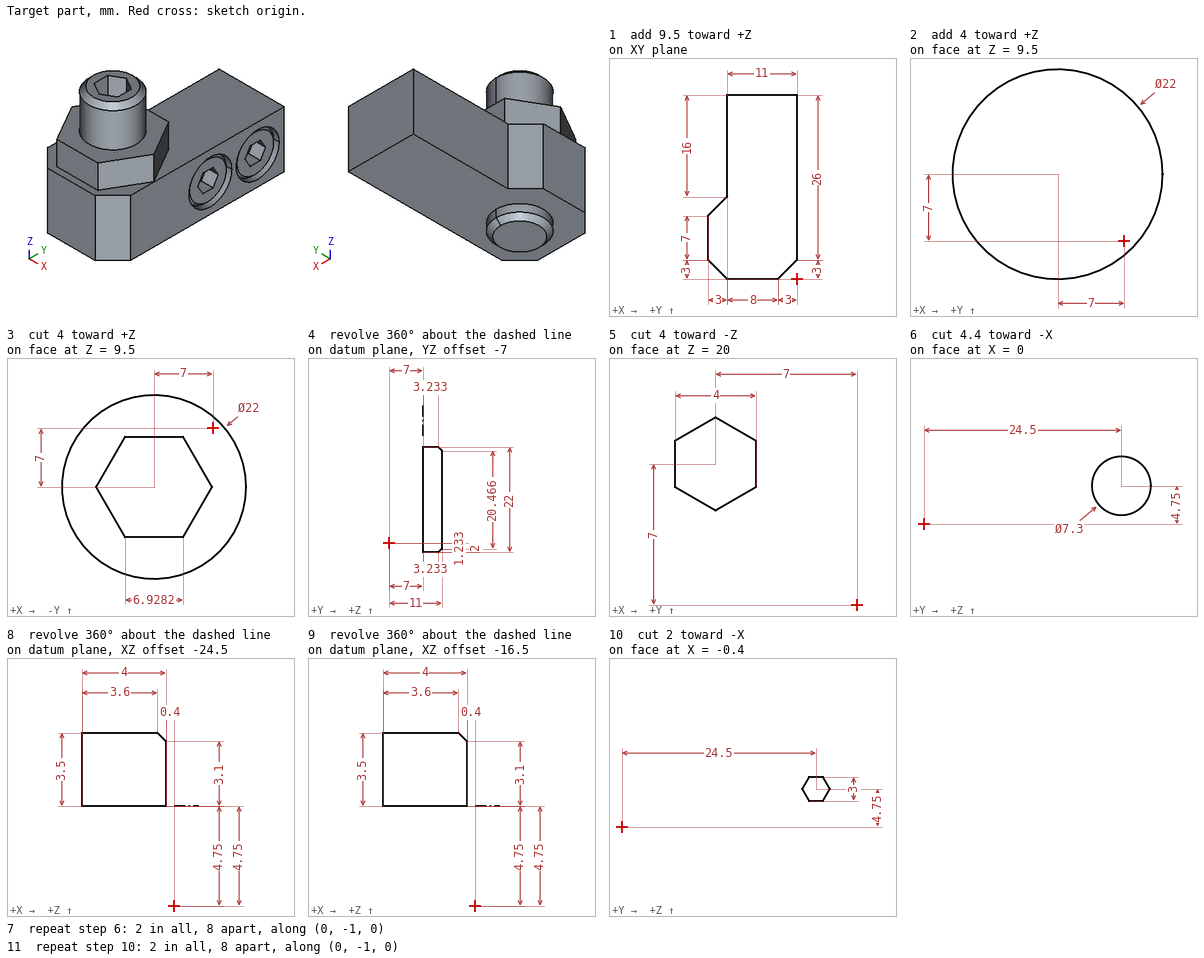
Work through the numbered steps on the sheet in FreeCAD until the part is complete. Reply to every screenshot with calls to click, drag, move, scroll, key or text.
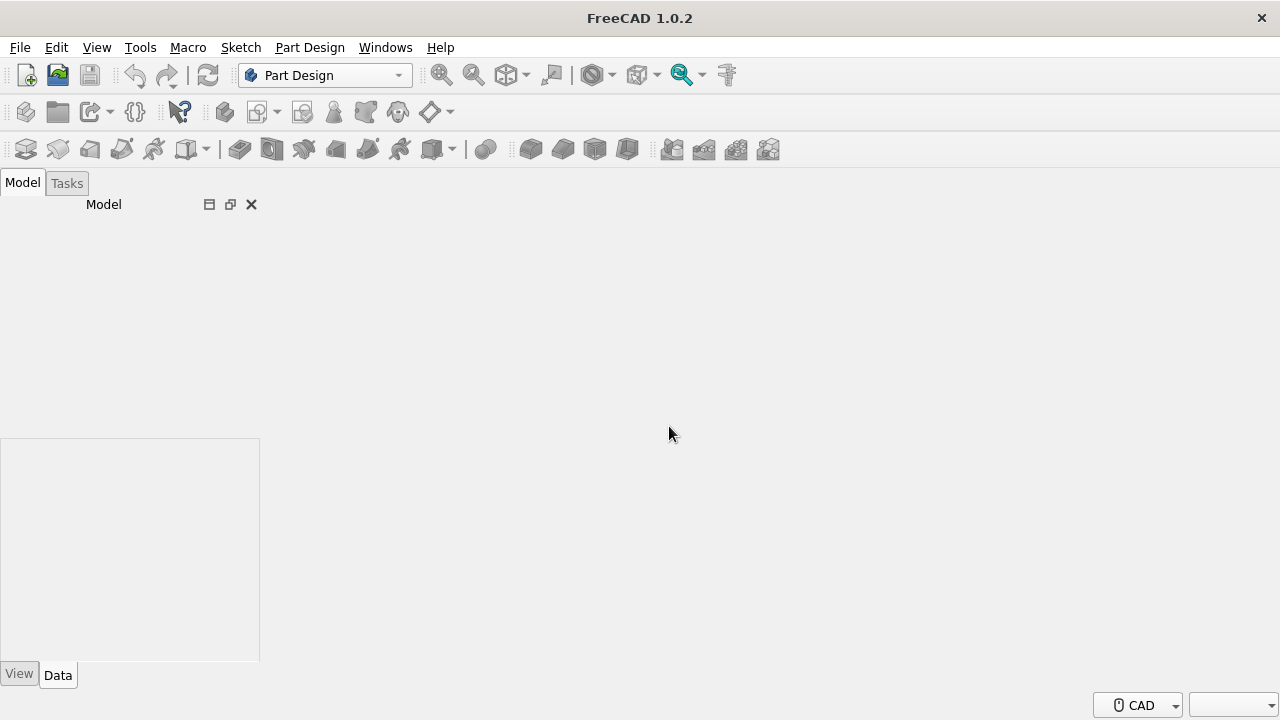
click(26, 76)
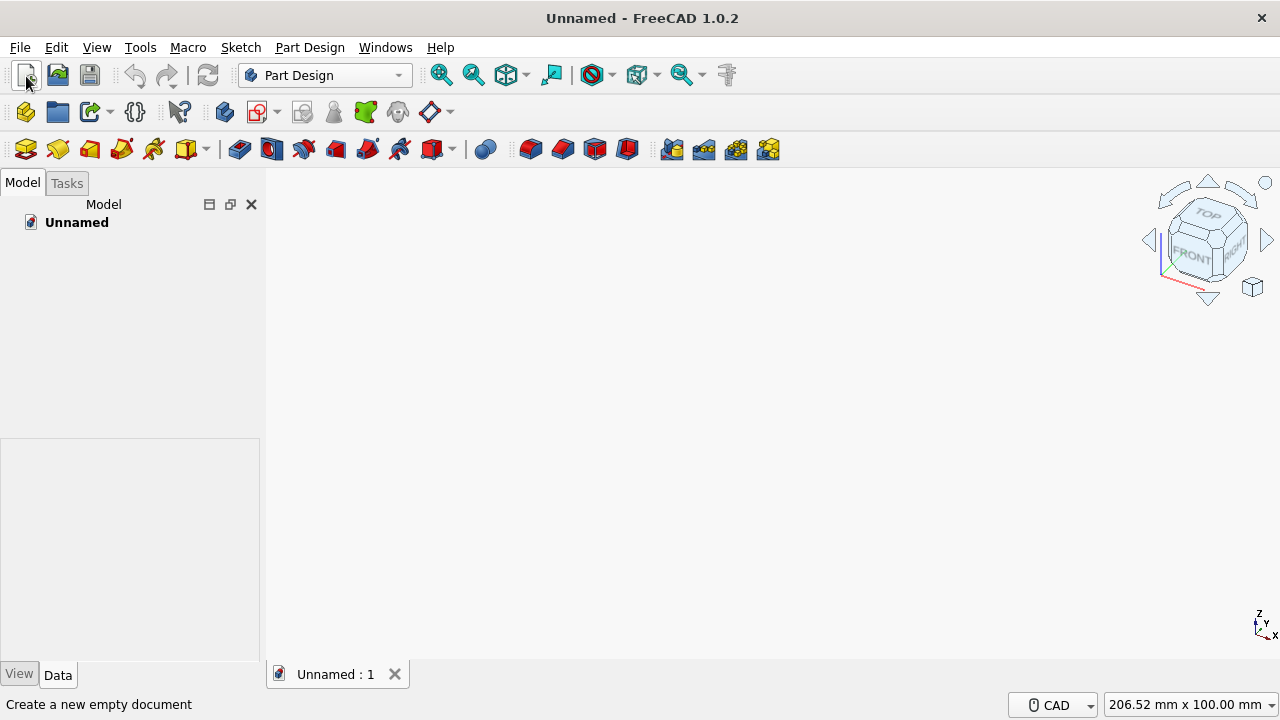
click(258, 112)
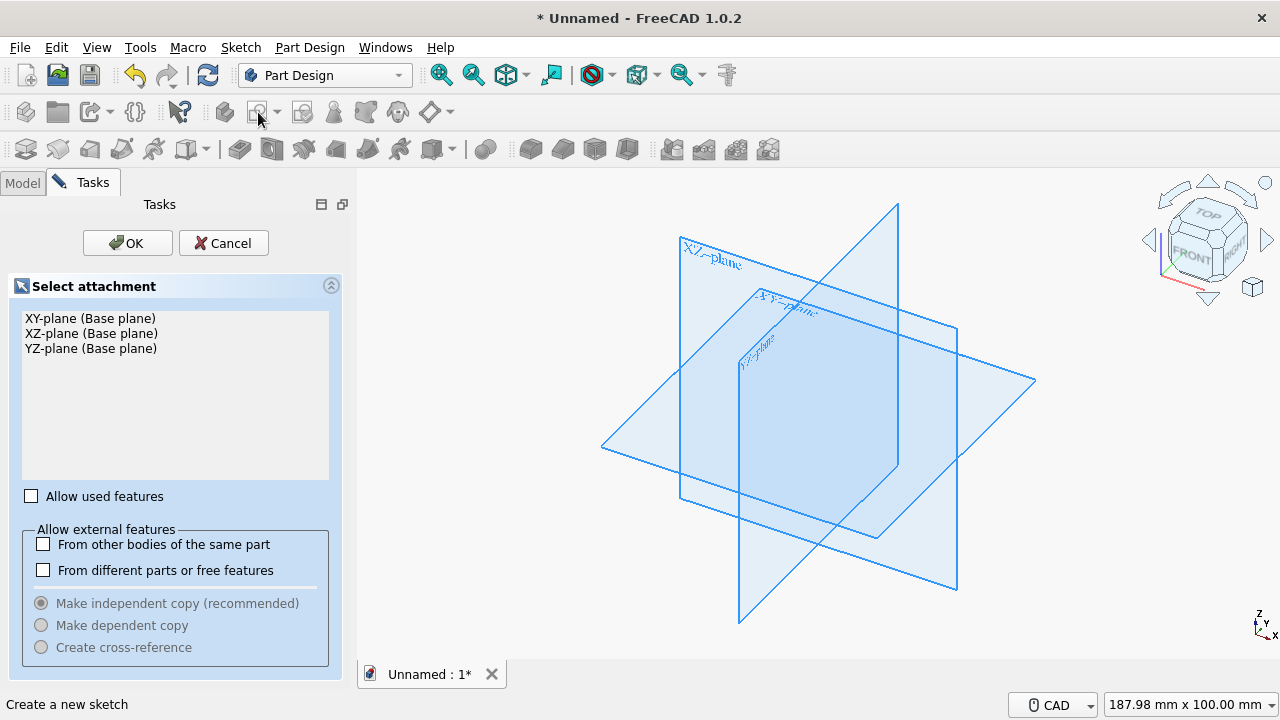
click(82, 318)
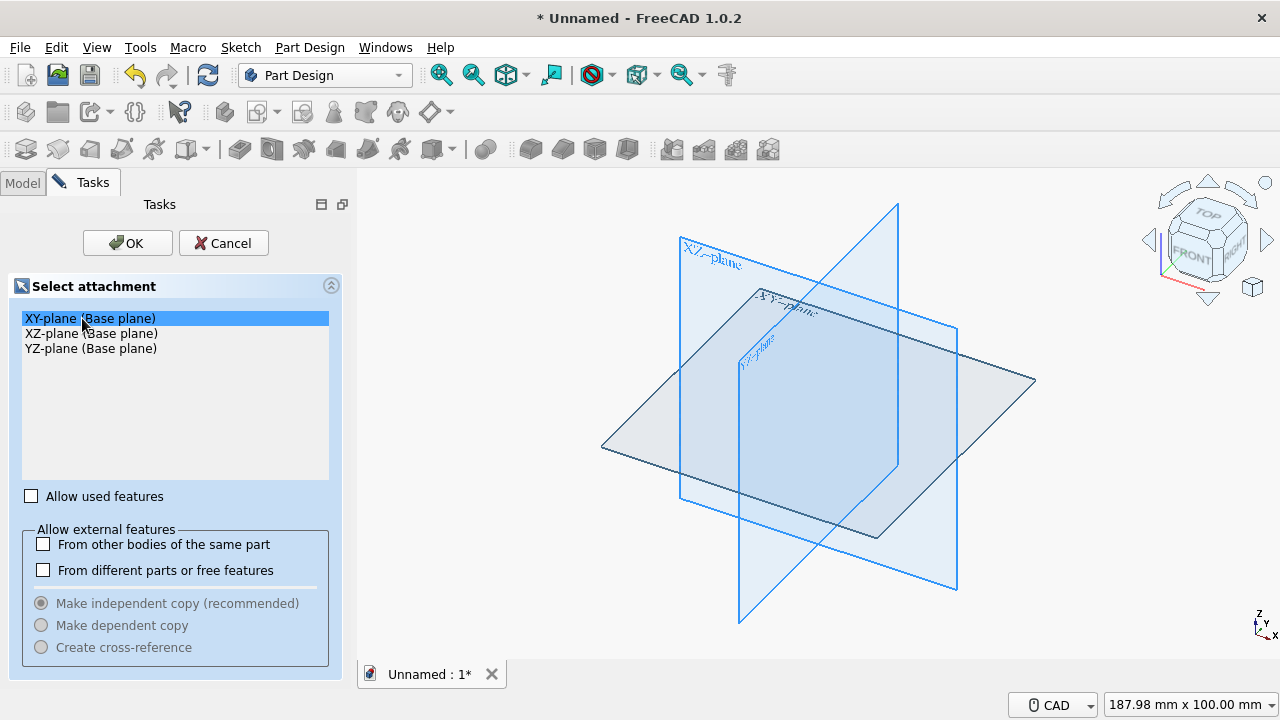
click(128, 243)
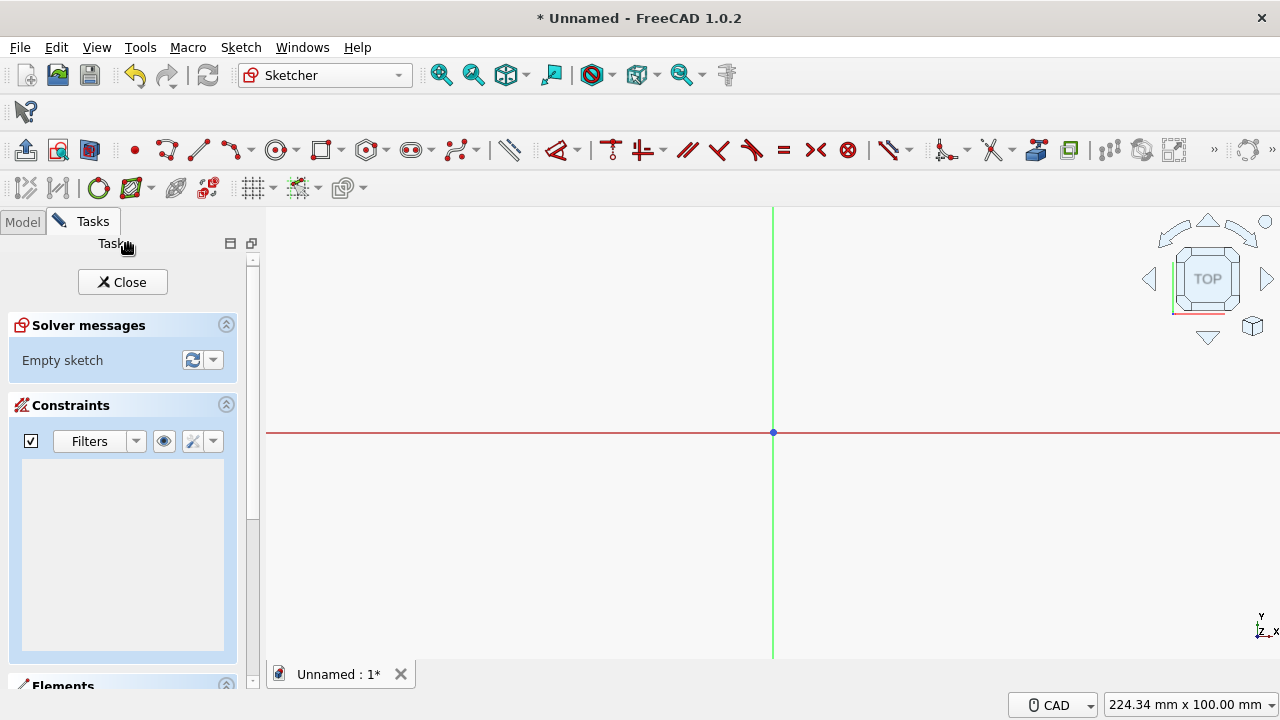
scroll(771, 314, up, 4)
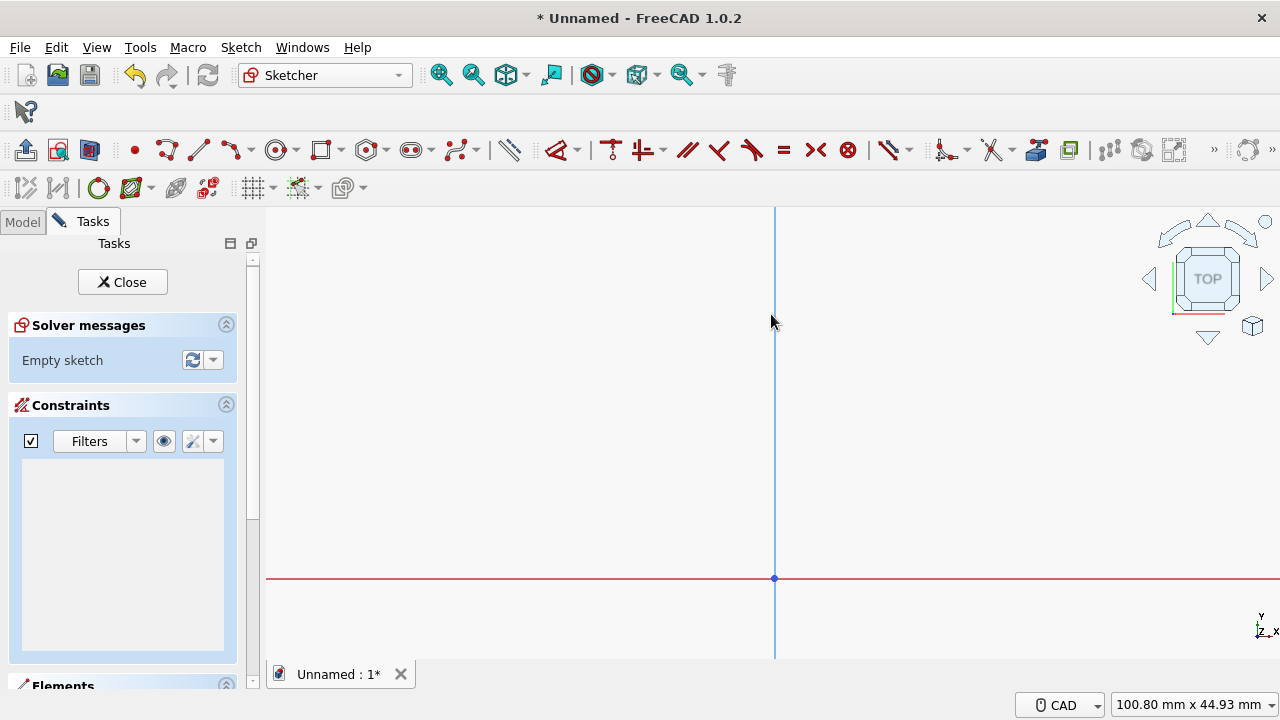
key(g)
key(m)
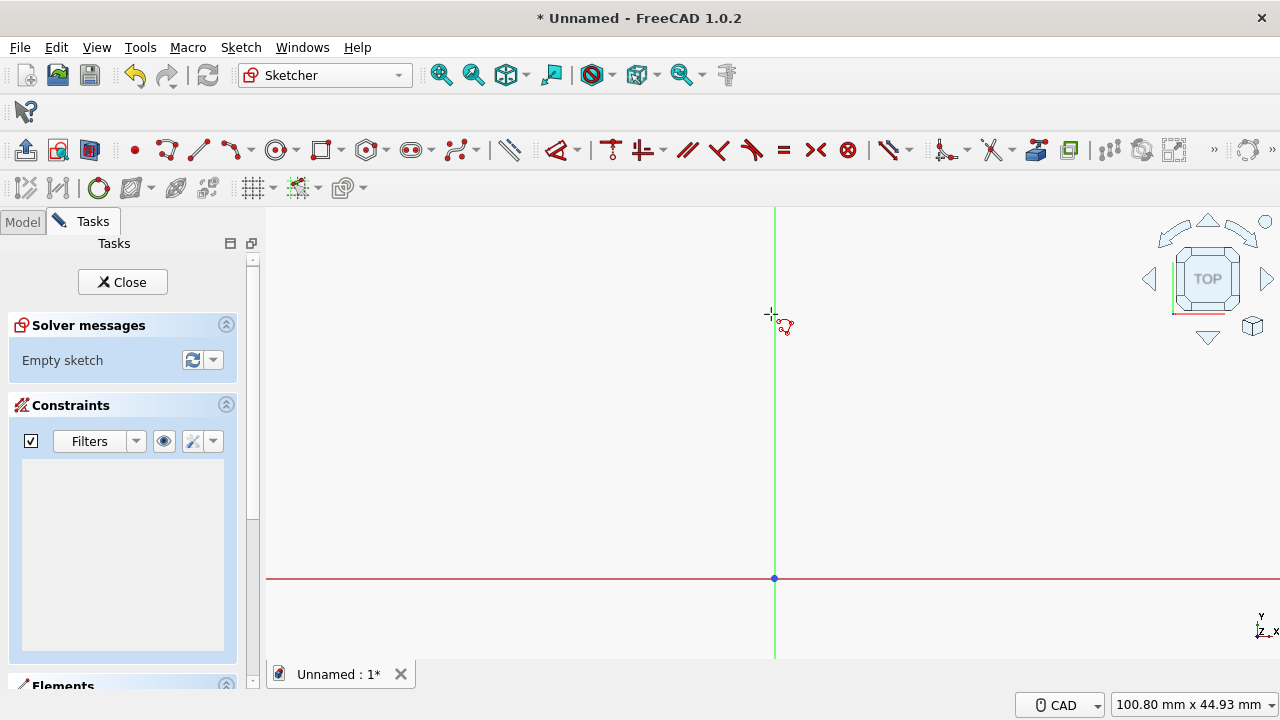
click(745, 579)
click(775, 548)
click(766, 287)
click(664, 287)
click(664, 448)
click(634, 478)
click(634, 548)
click(664, 570)
click(745, 579)
key(Escape)
key(Escape)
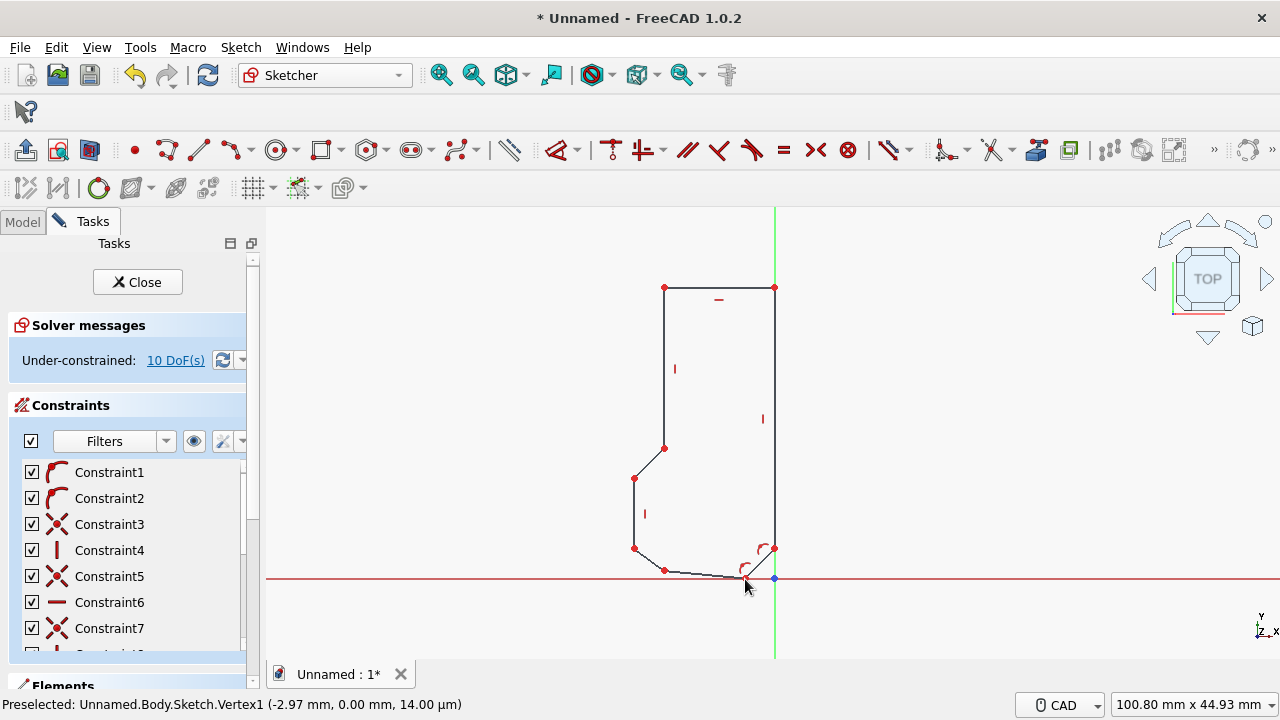
click(721, 576)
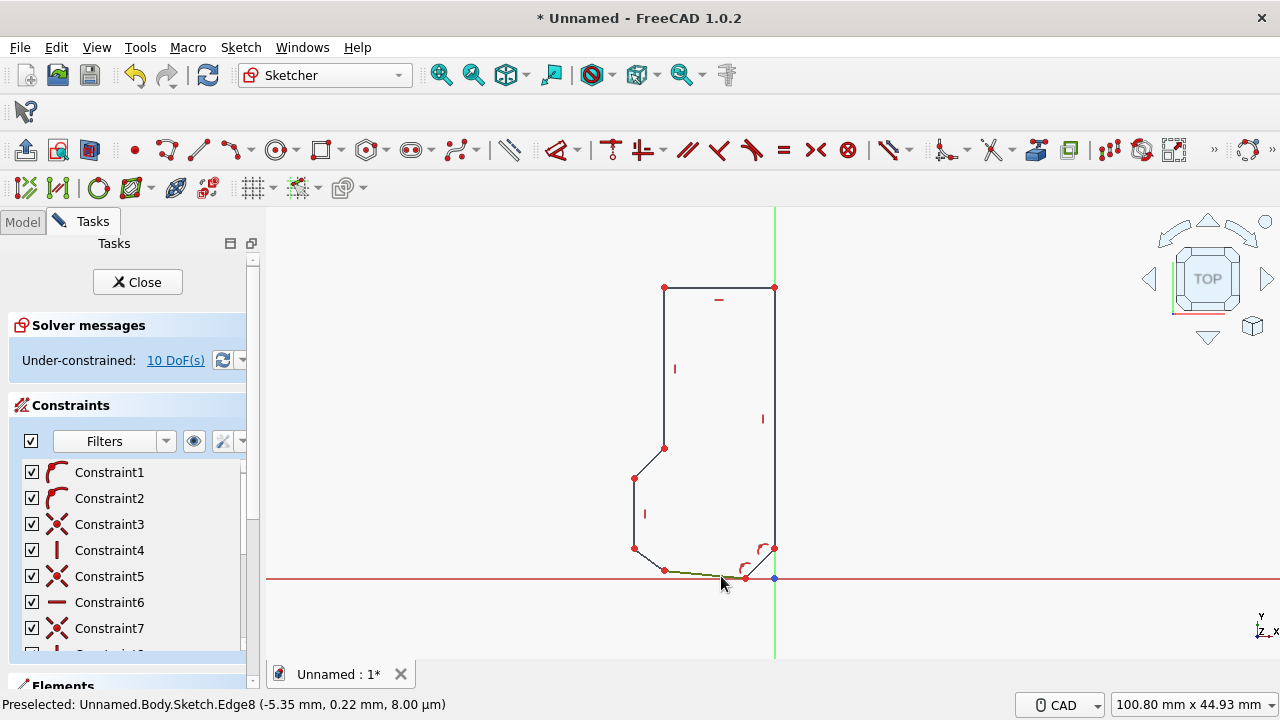
key(h)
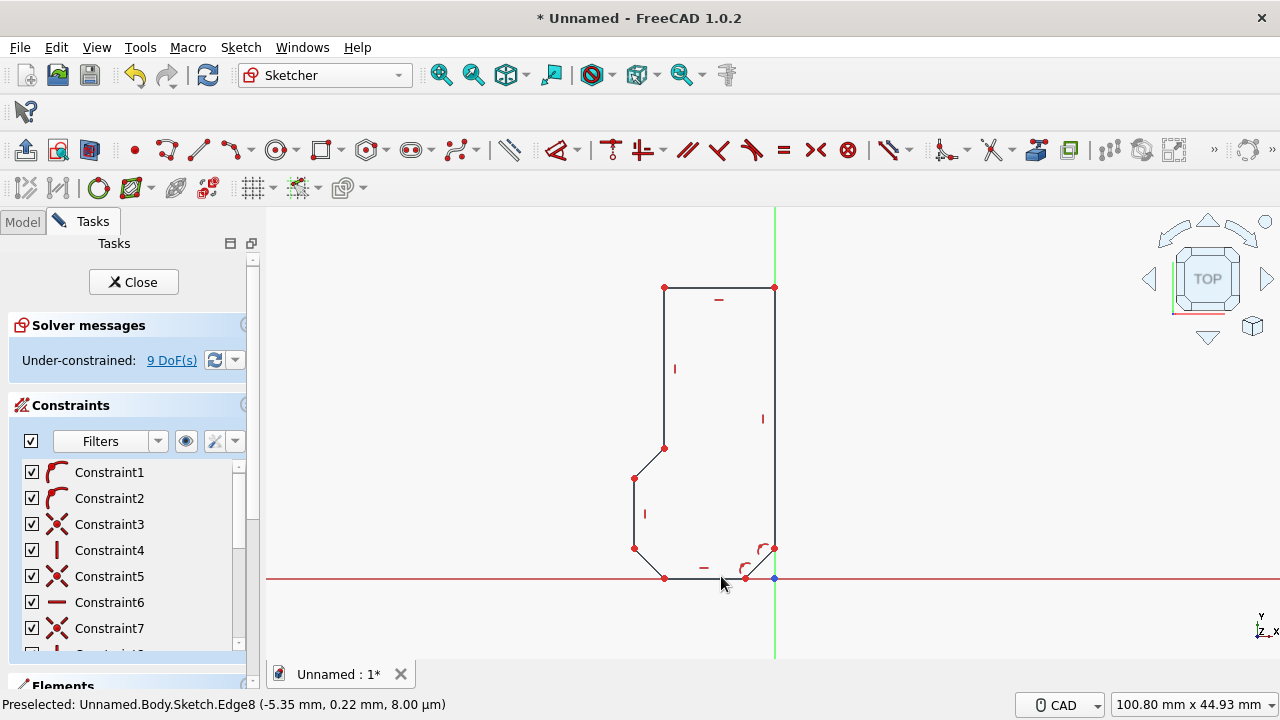
click(634, 500)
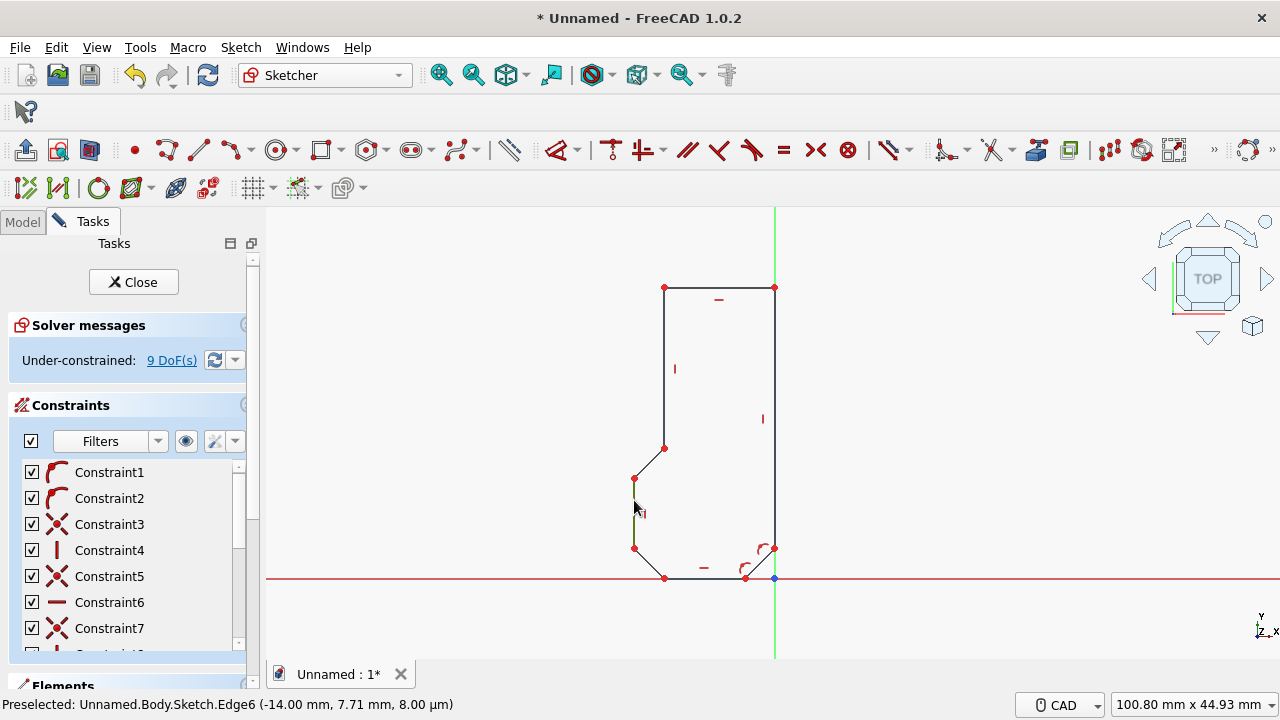
key(i)